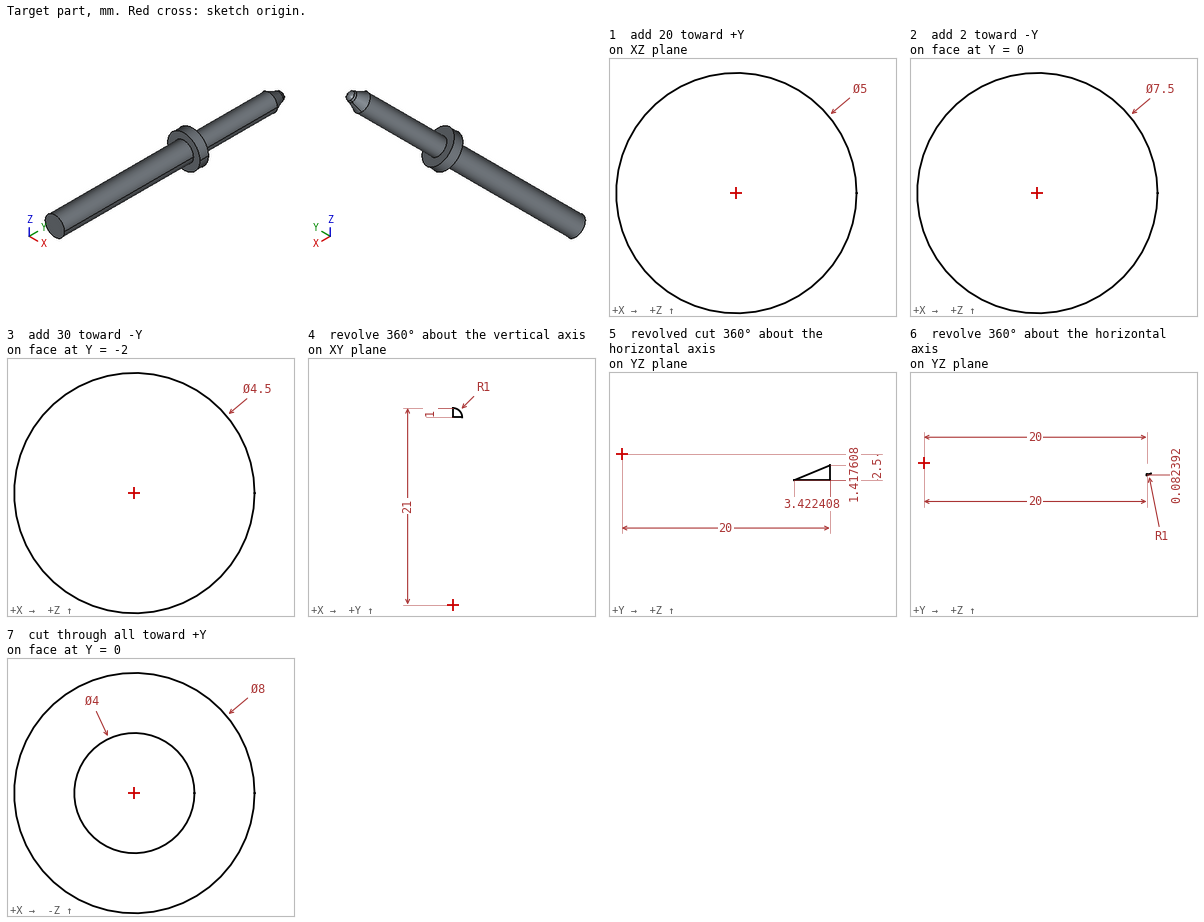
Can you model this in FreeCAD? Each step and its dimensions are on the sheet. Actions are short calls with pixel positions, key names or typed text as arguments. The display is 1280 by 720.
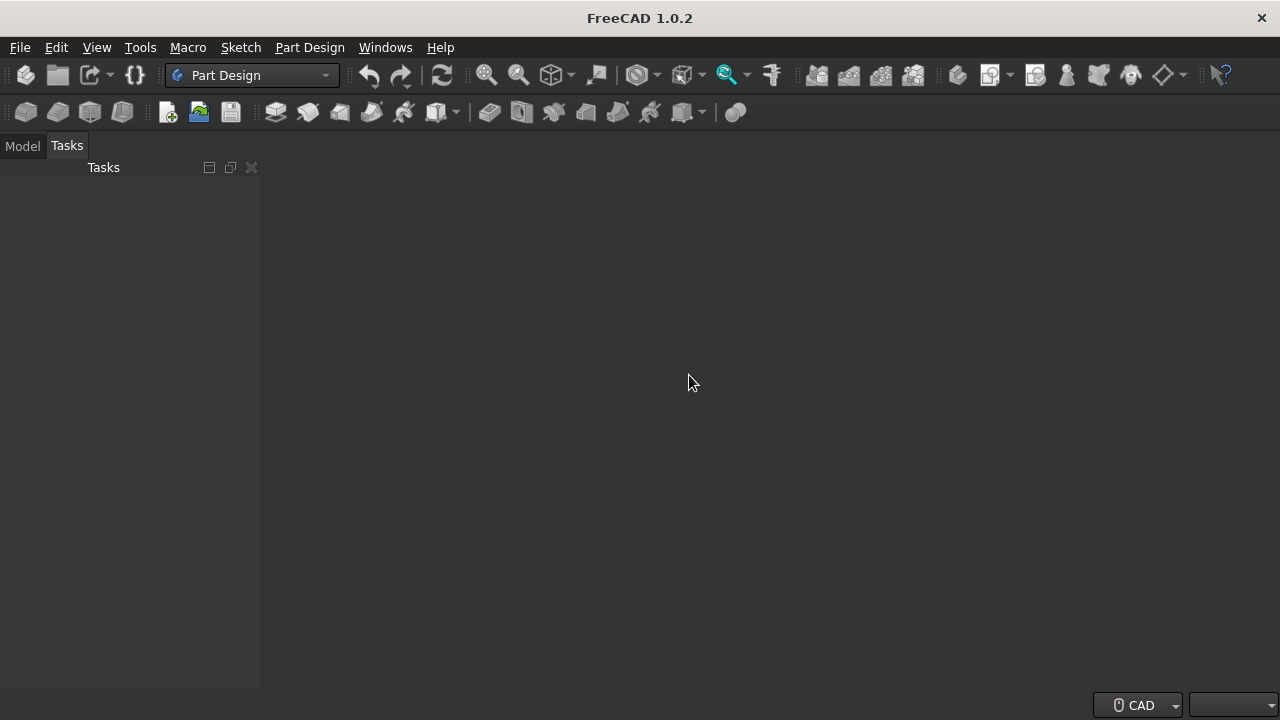
click(168, 112)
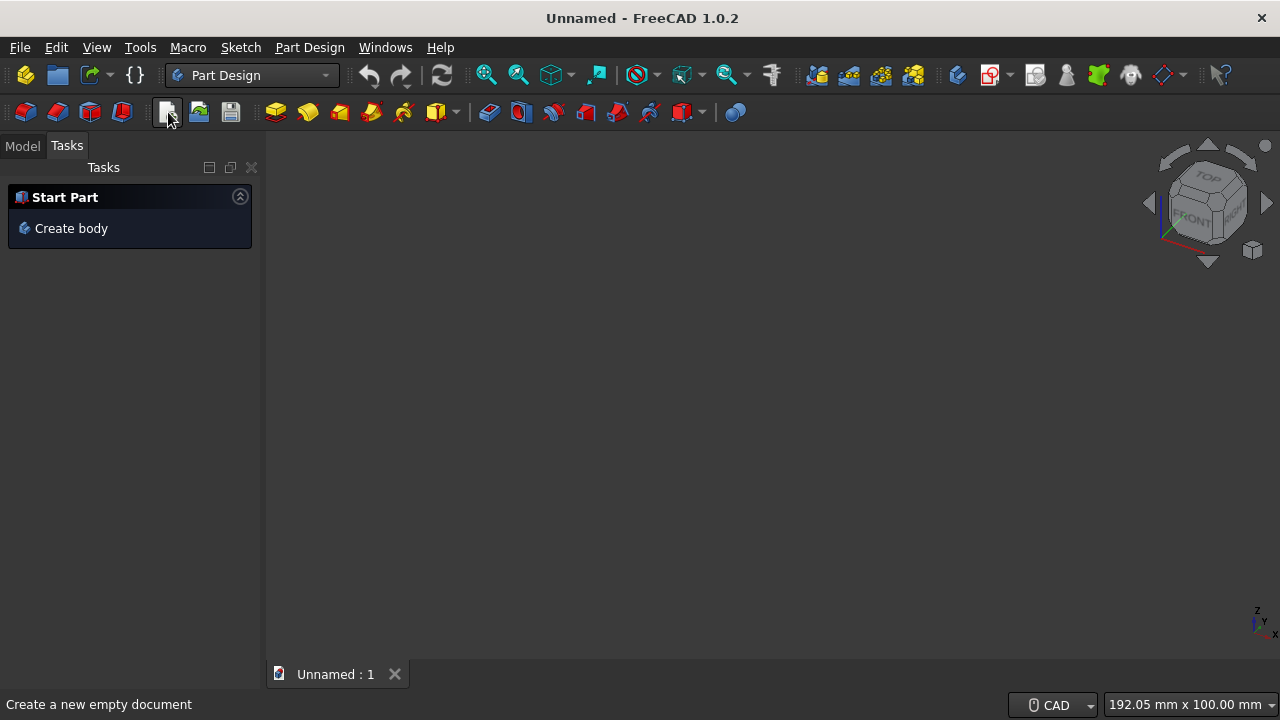
click(990, 76)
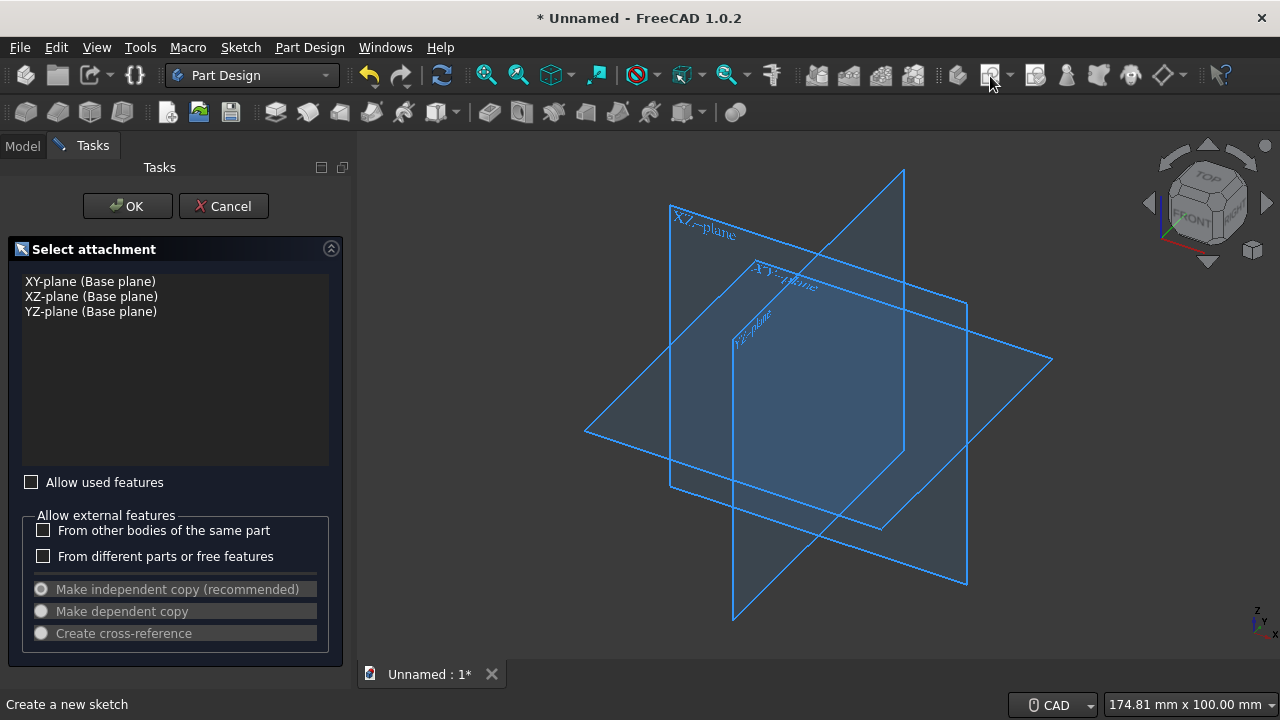
click(82, 296)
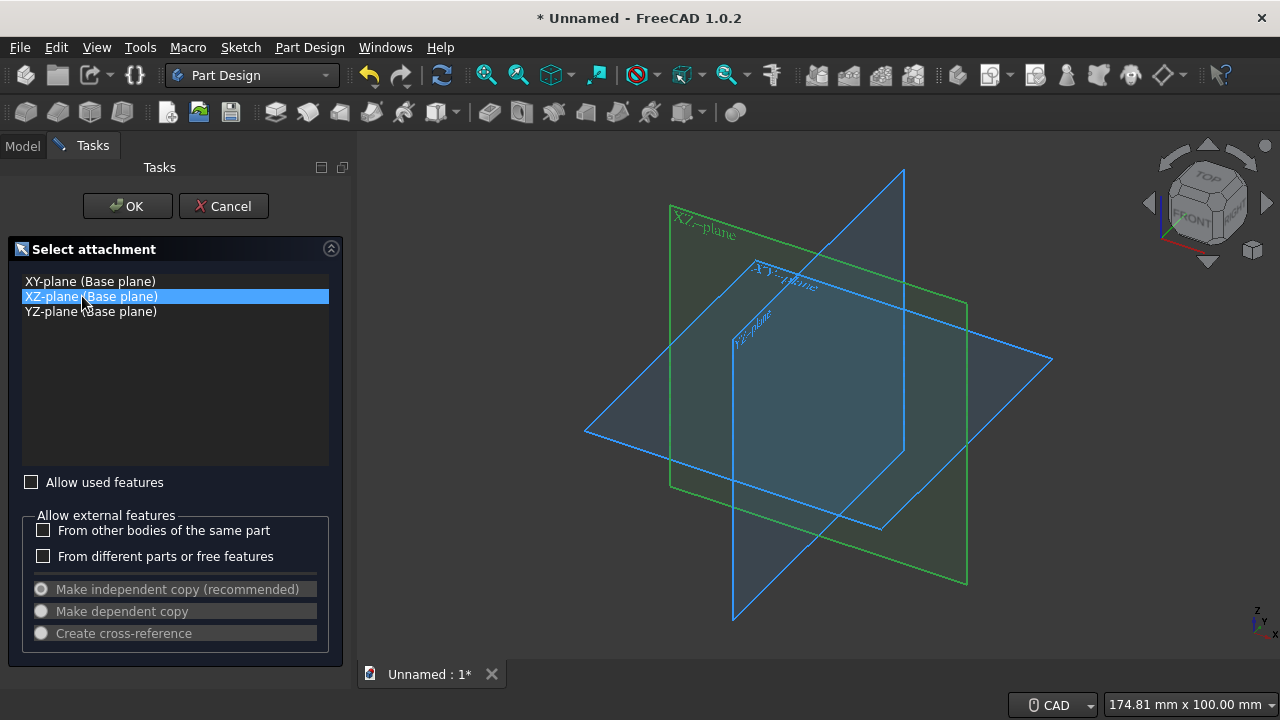
click(128, 206)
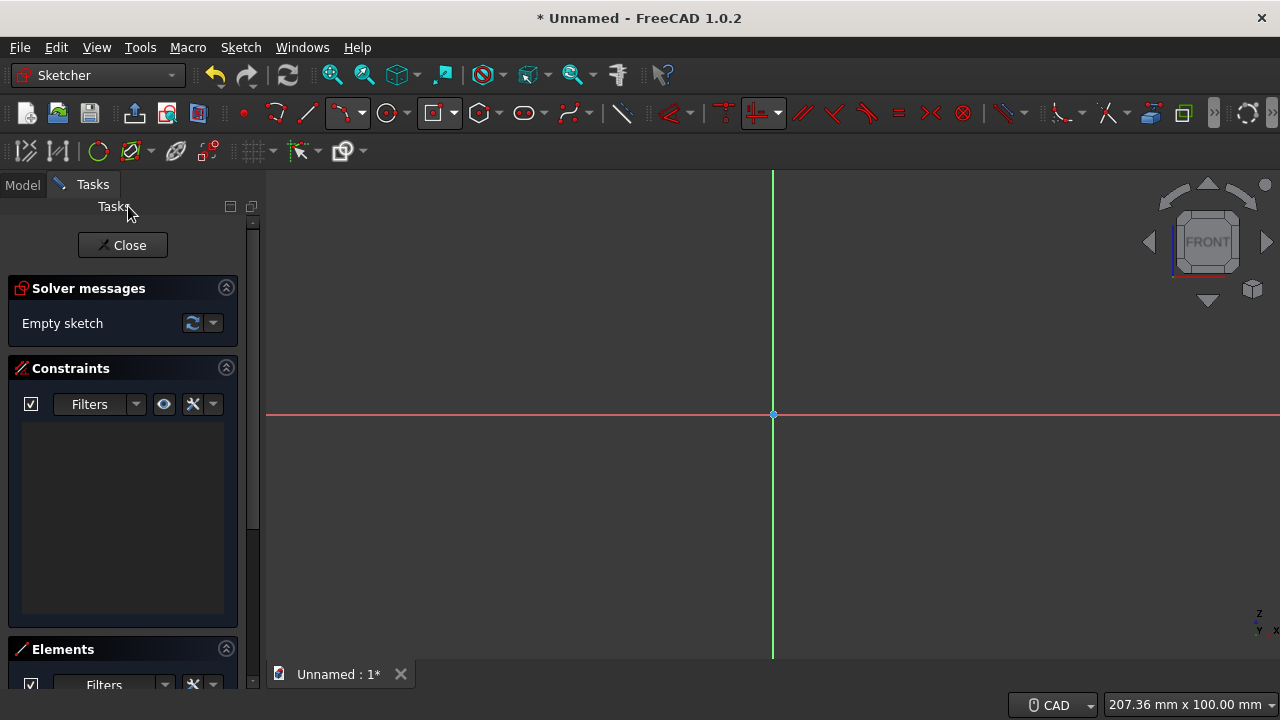
scroll(778, 415, up, 13)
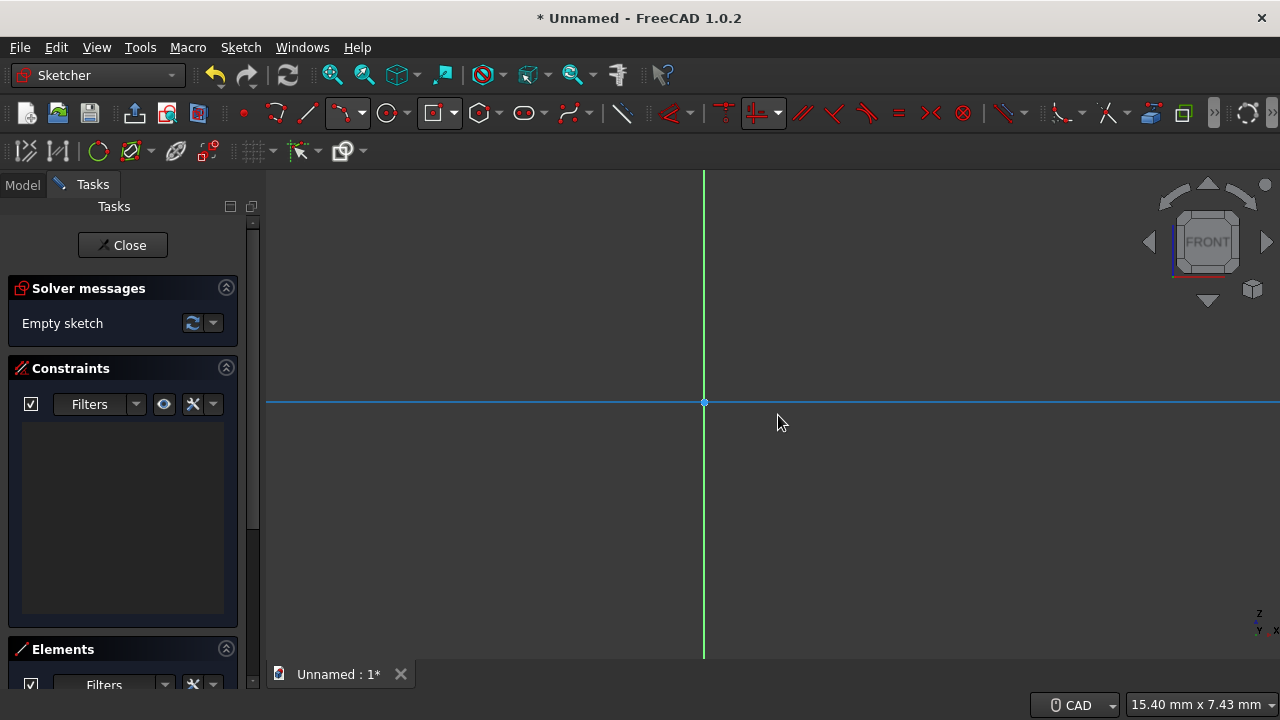
click(388, 114)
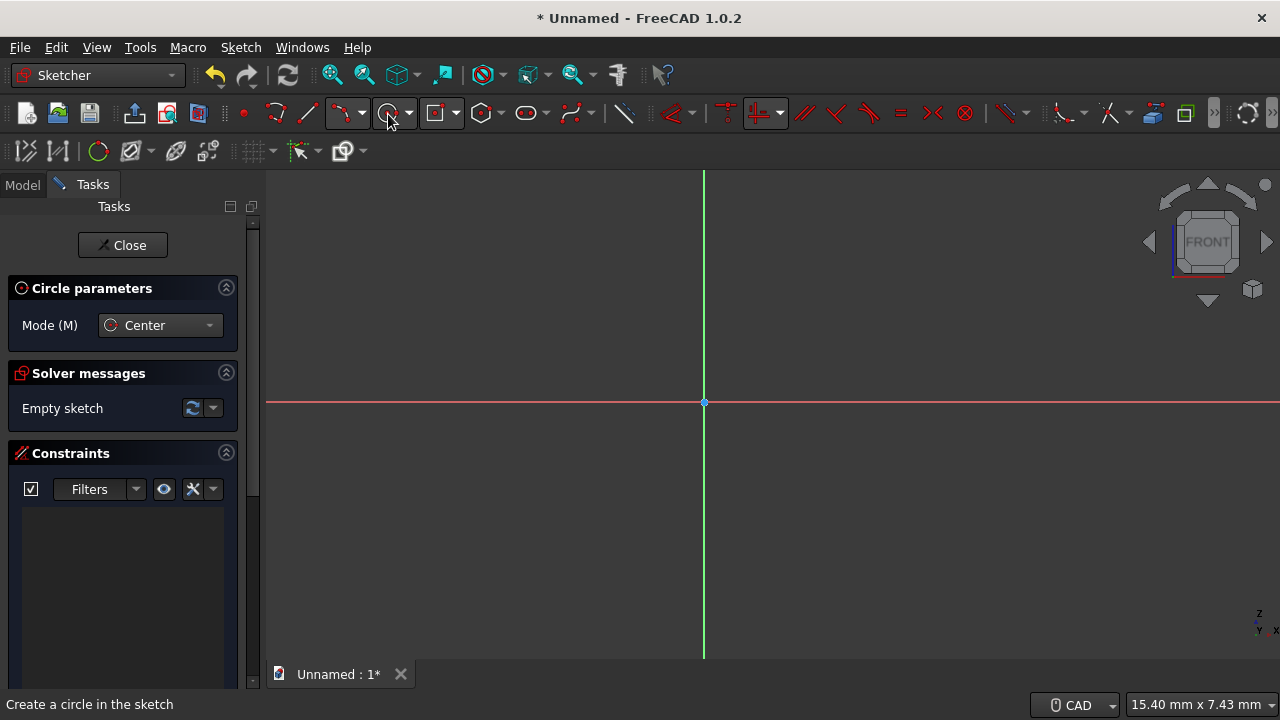
click(704, 402)
click(821, 286)
key(Escape)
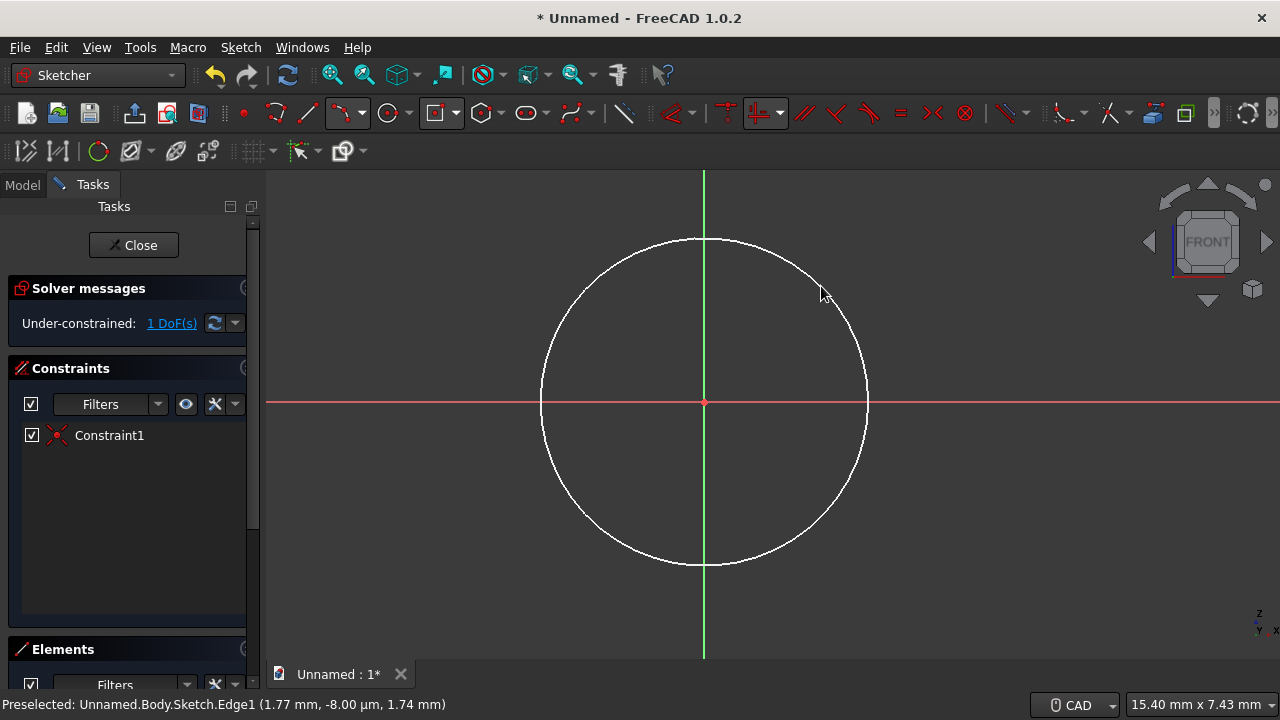
key(d)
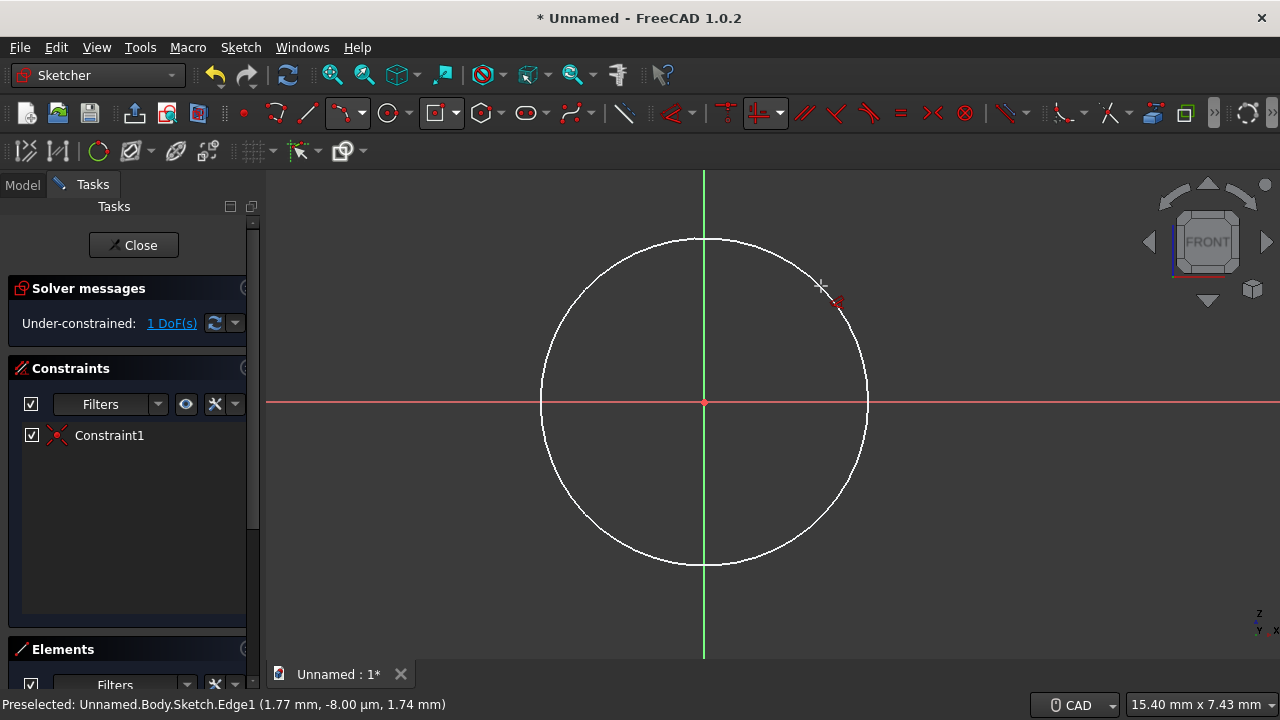
click(820, 286)
click(843, 263)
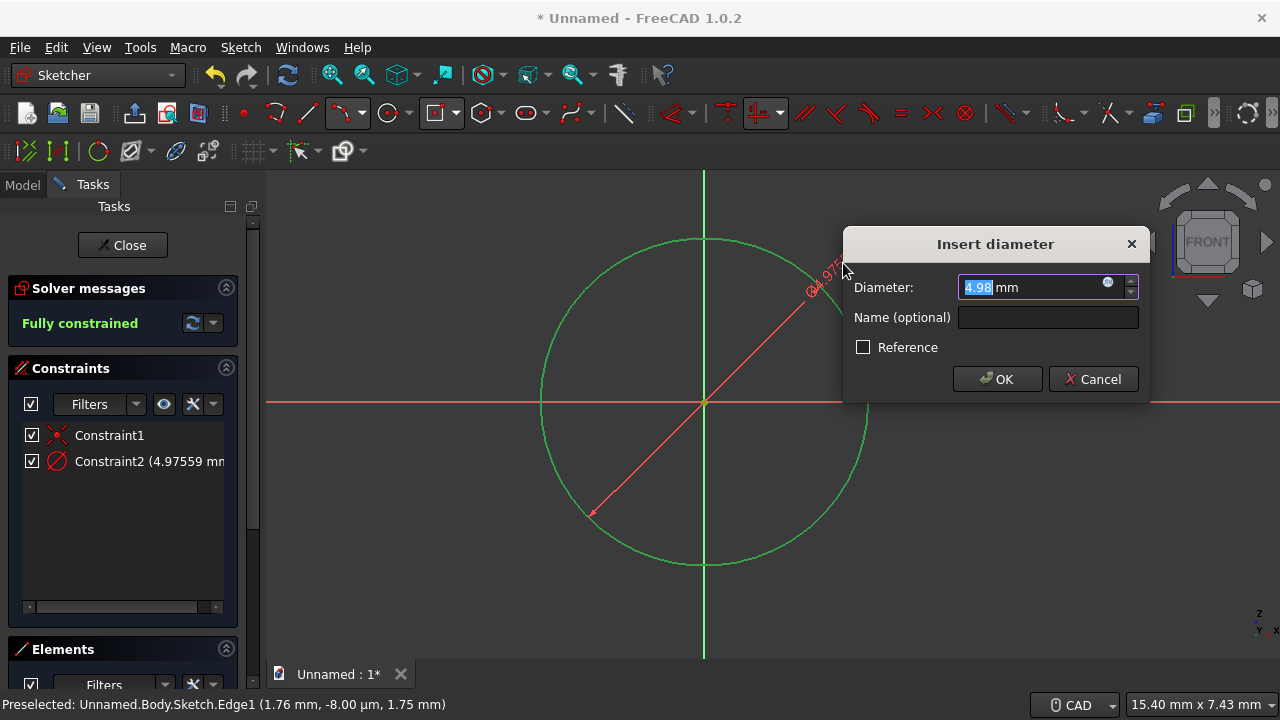
text(5)
key(Return)
key(Escape)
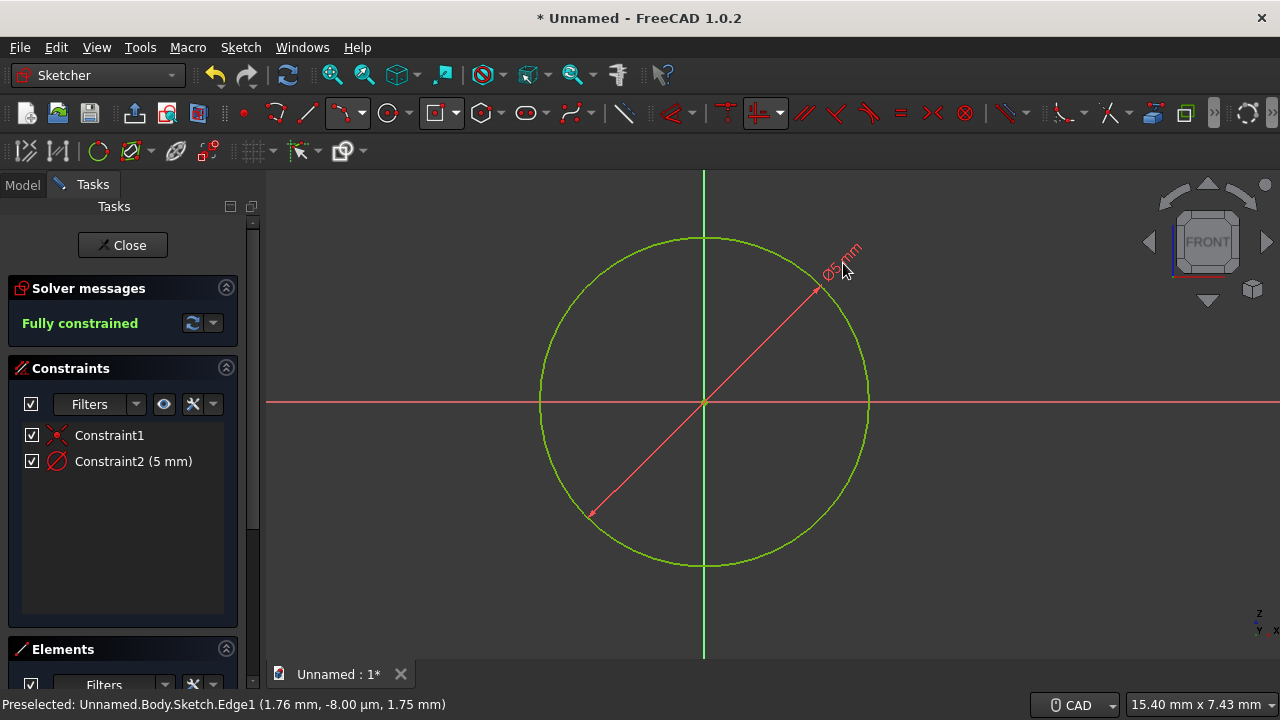
click(123, 245)